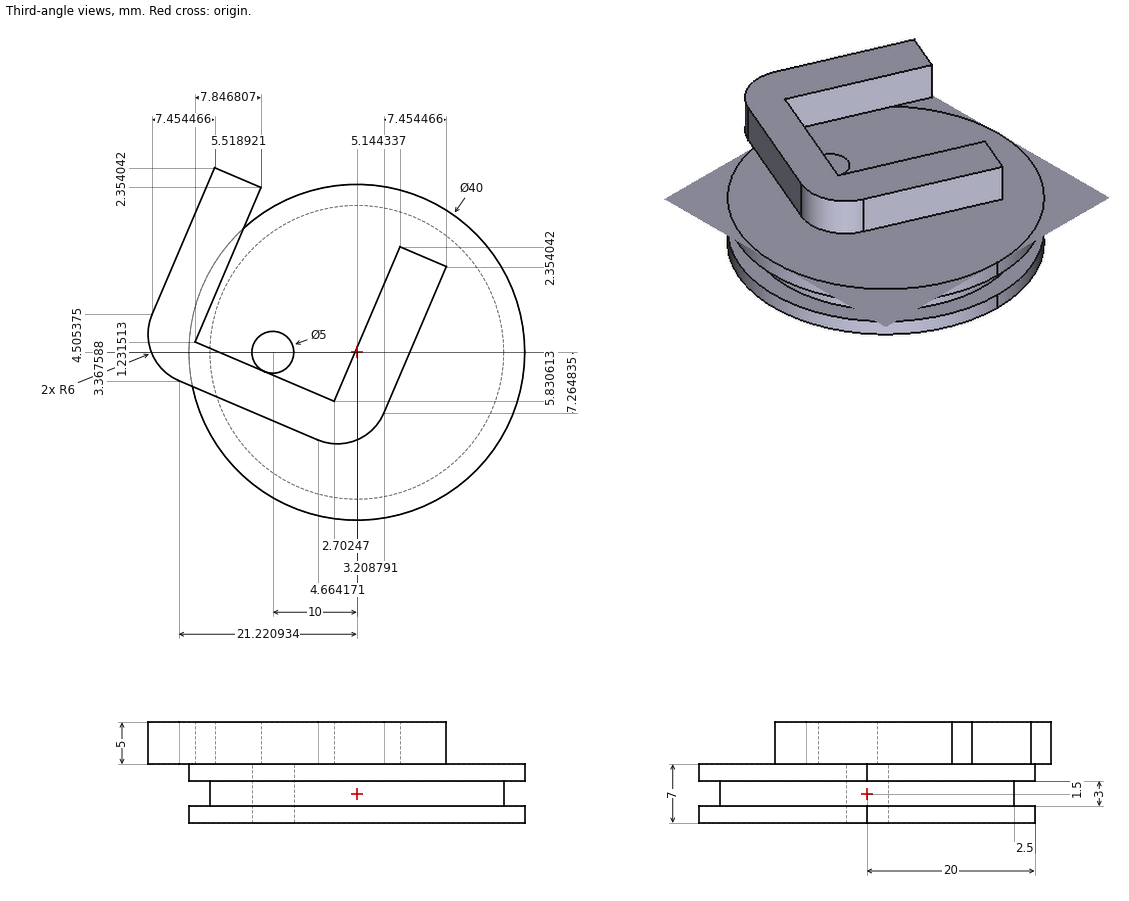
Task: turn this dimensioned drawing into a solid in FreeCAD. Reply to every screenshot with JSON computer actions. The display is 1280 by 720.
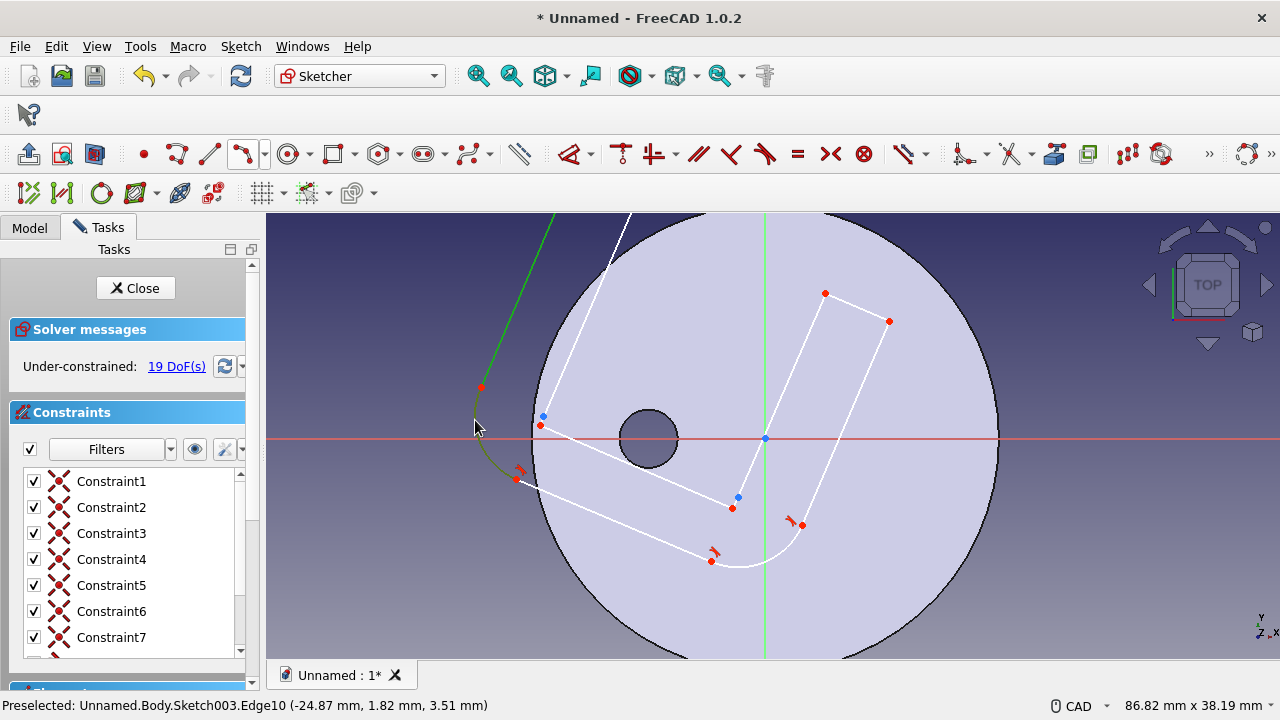
{"action": "left_click", "coordinate": [765, 154]}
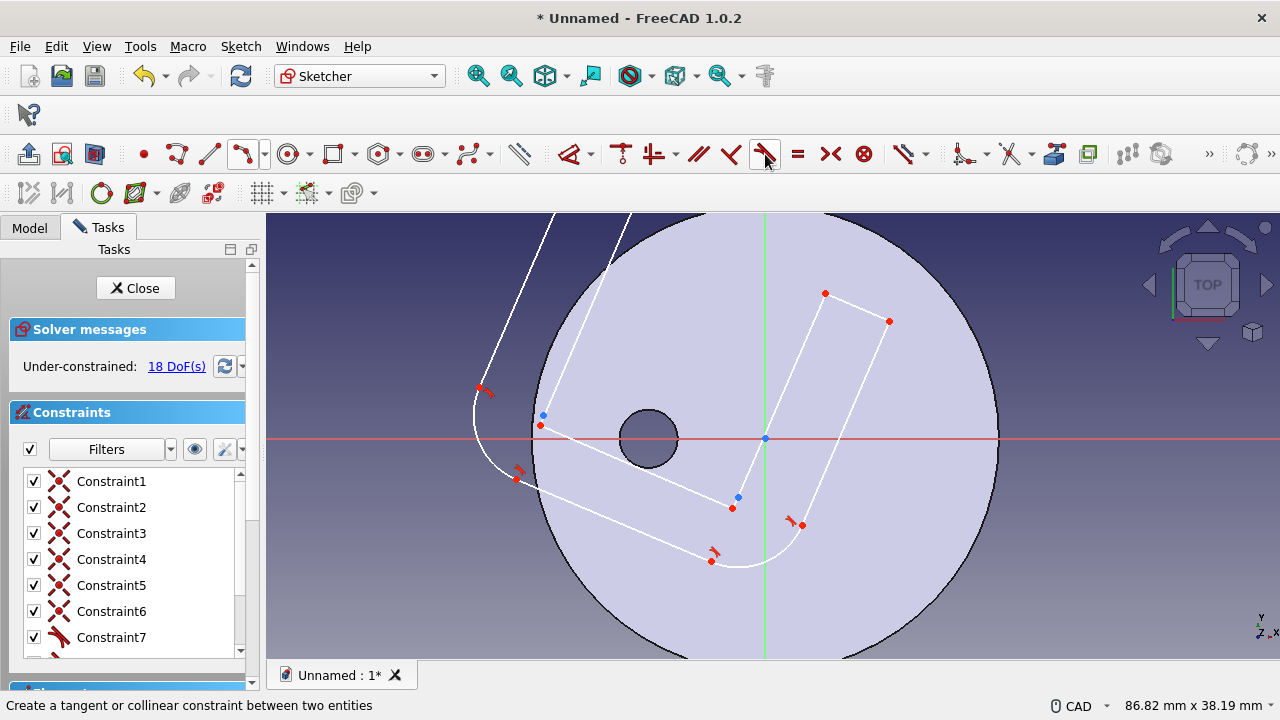
{"action": "left_click", "coordinate": [743, 567]}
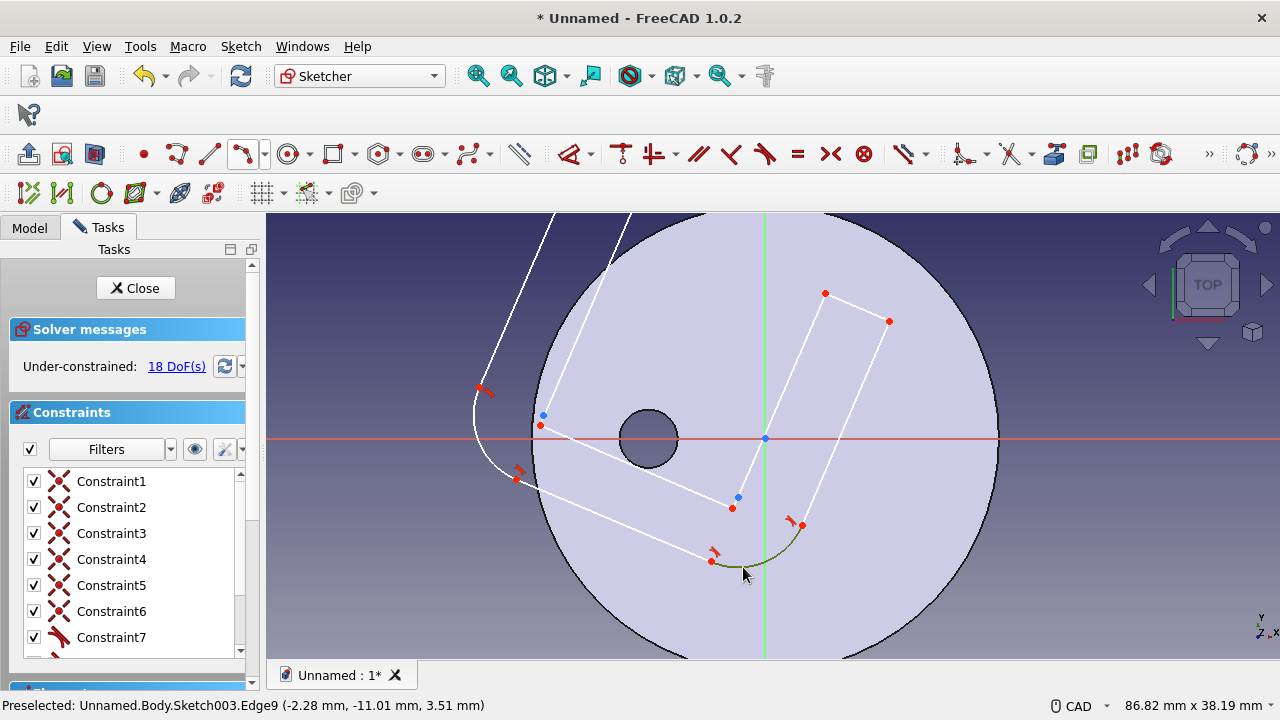
{"action": "left_click", "coordinate": [474, 420]}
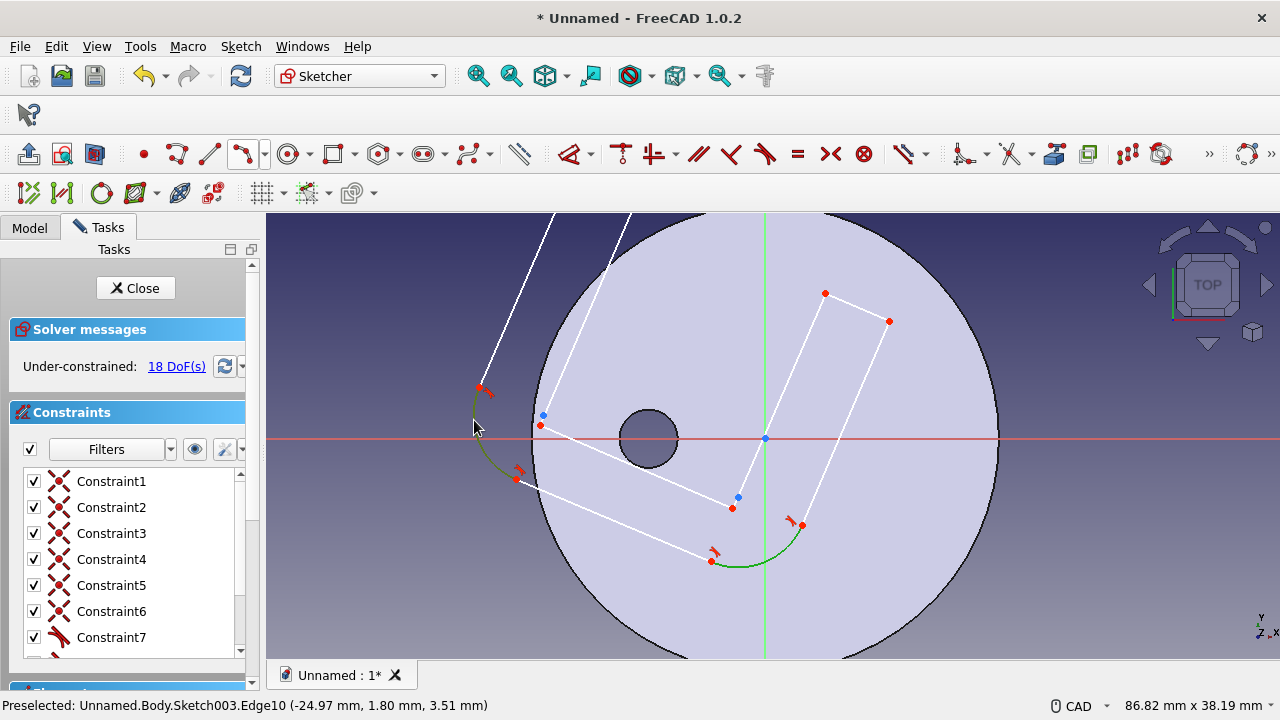
{"action": "left_click", "coordinate": [798, 154]}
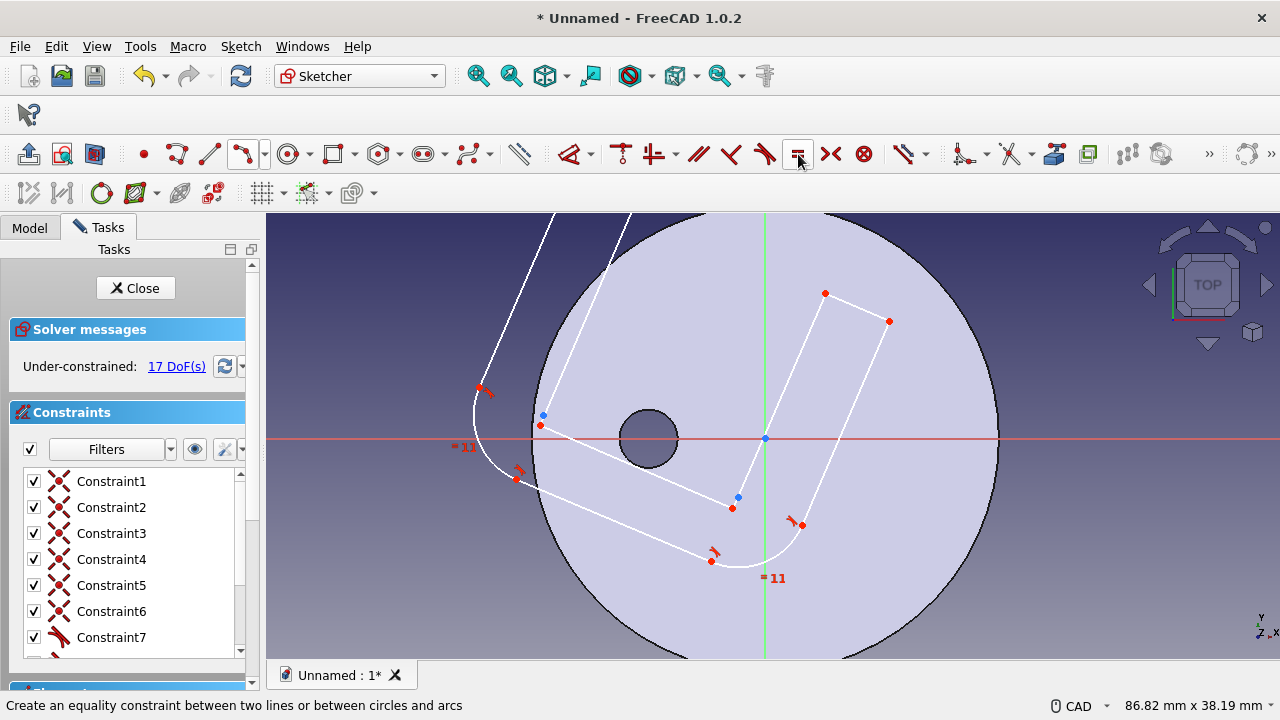
{"action": "left_click", "coordinate": [568, 154]}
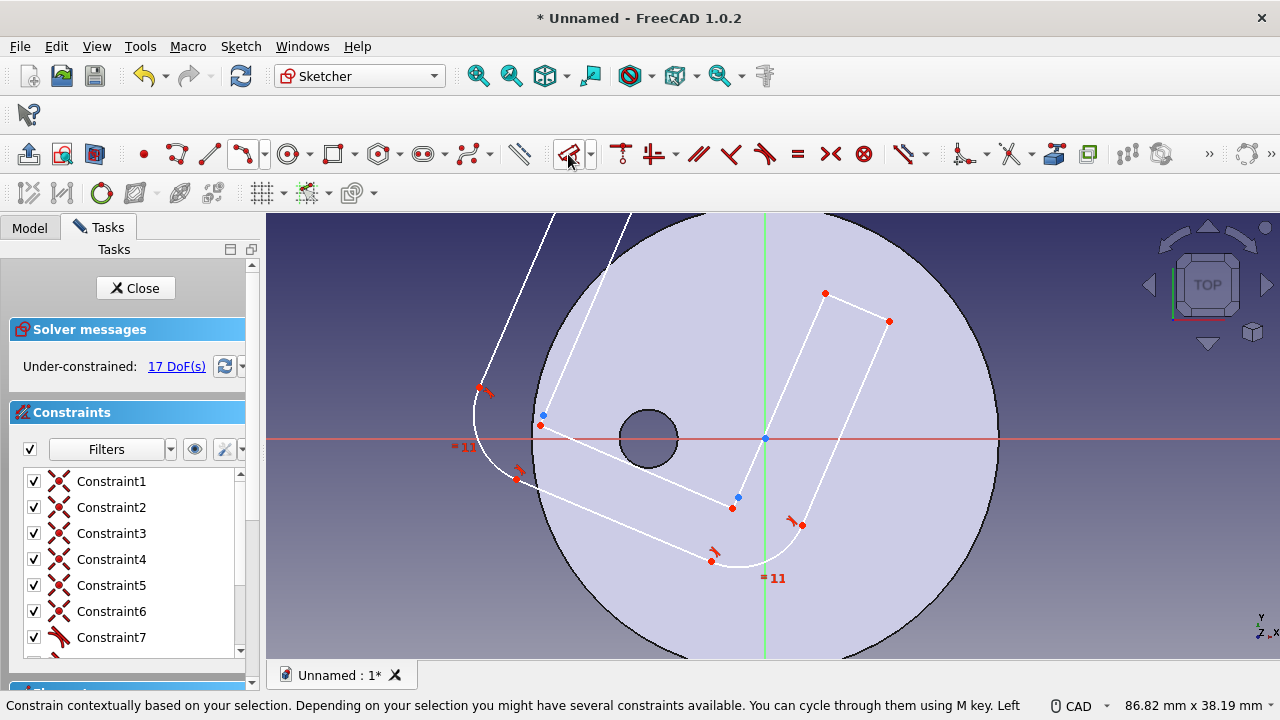
{"action": "left_click", "coordinate": [743, 567]}
{"action": "left_click", "coordinate": [745, 599]}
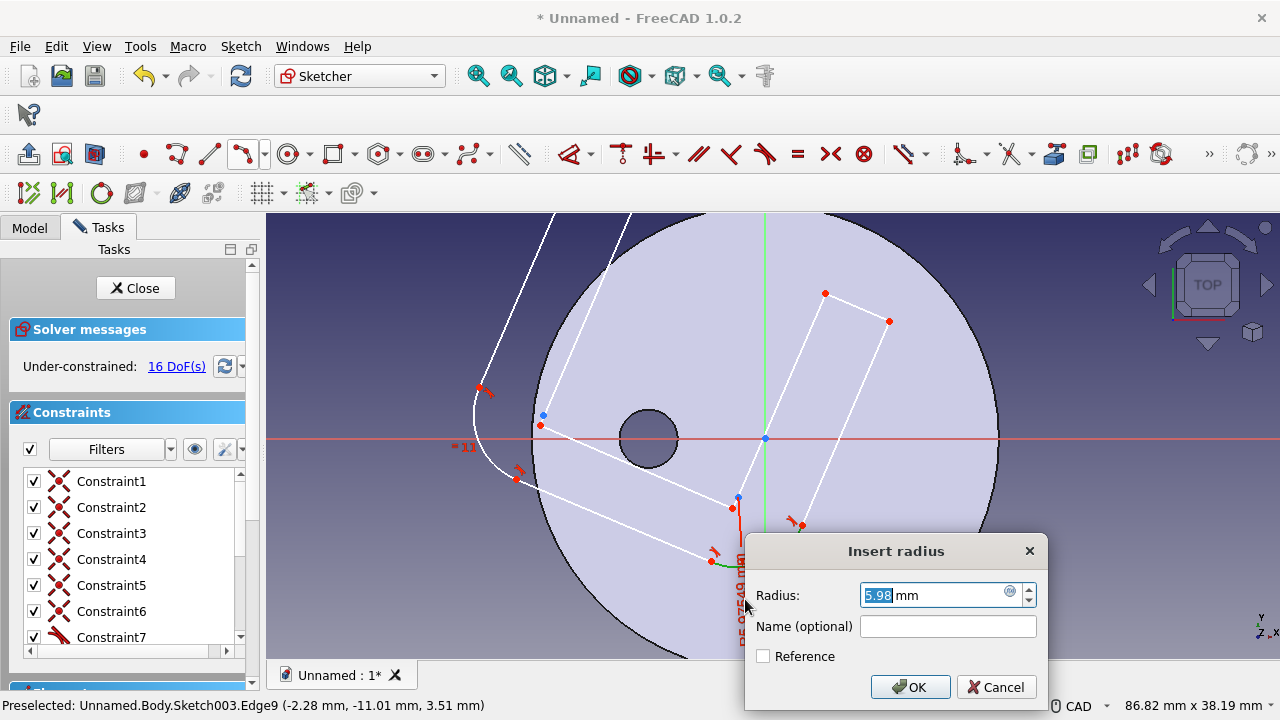
{"action": "type", "text": "6"}
{"action": "key", "text": "Return"}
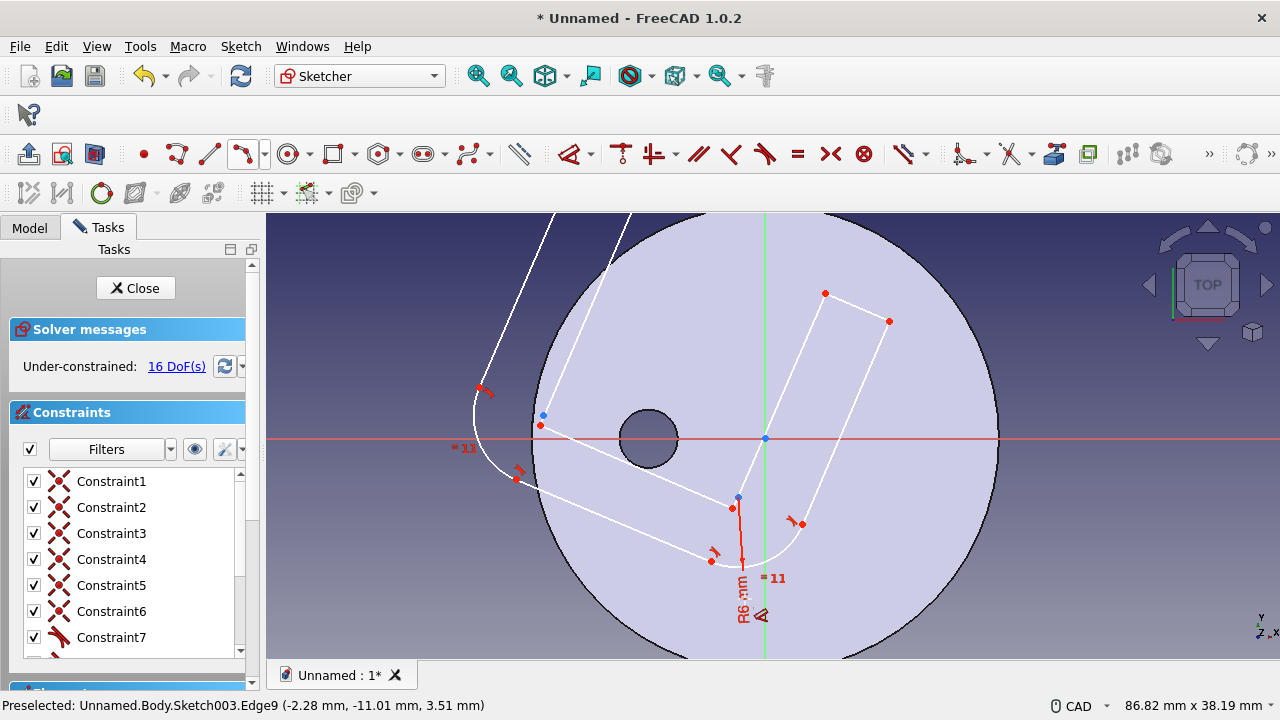
{"action": "scroll", "coordinate": [733, 509], "scroll_direction": "up", "scroll_amount": 2}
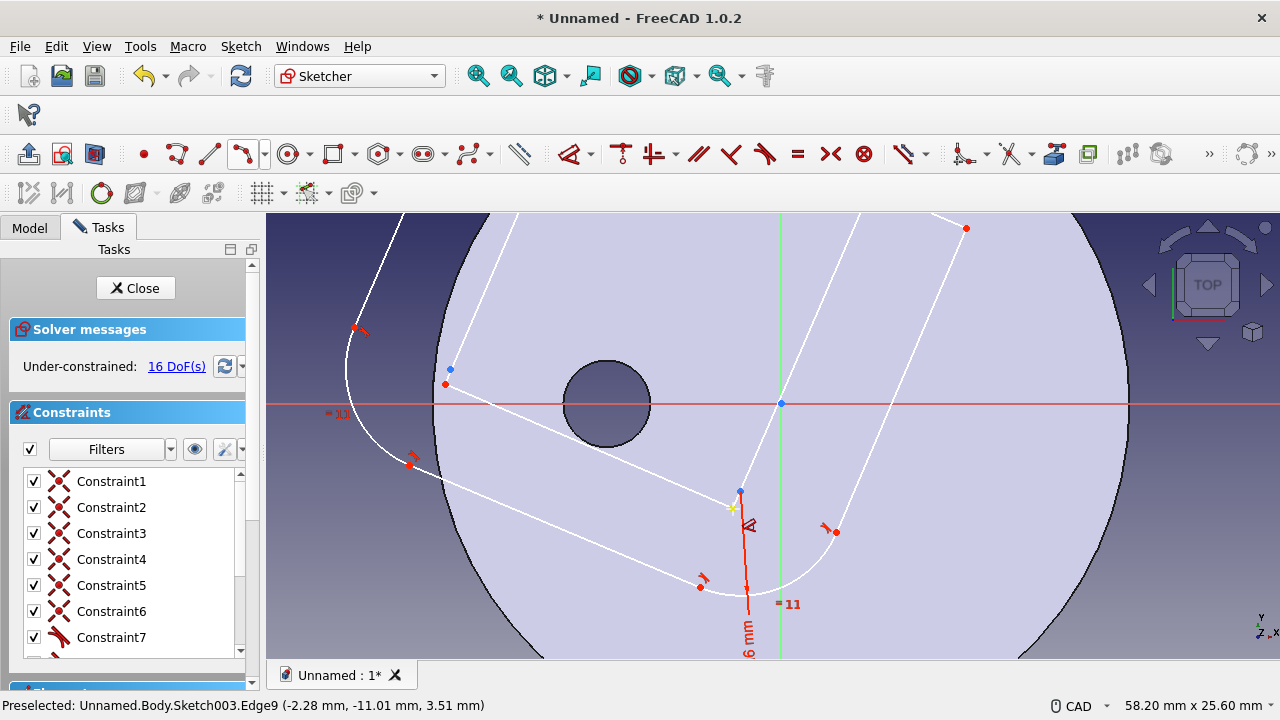
{"action": "left_click", "coordinate": [733, 508]}
{"action": "left_click", "coordinate": [757, 542]}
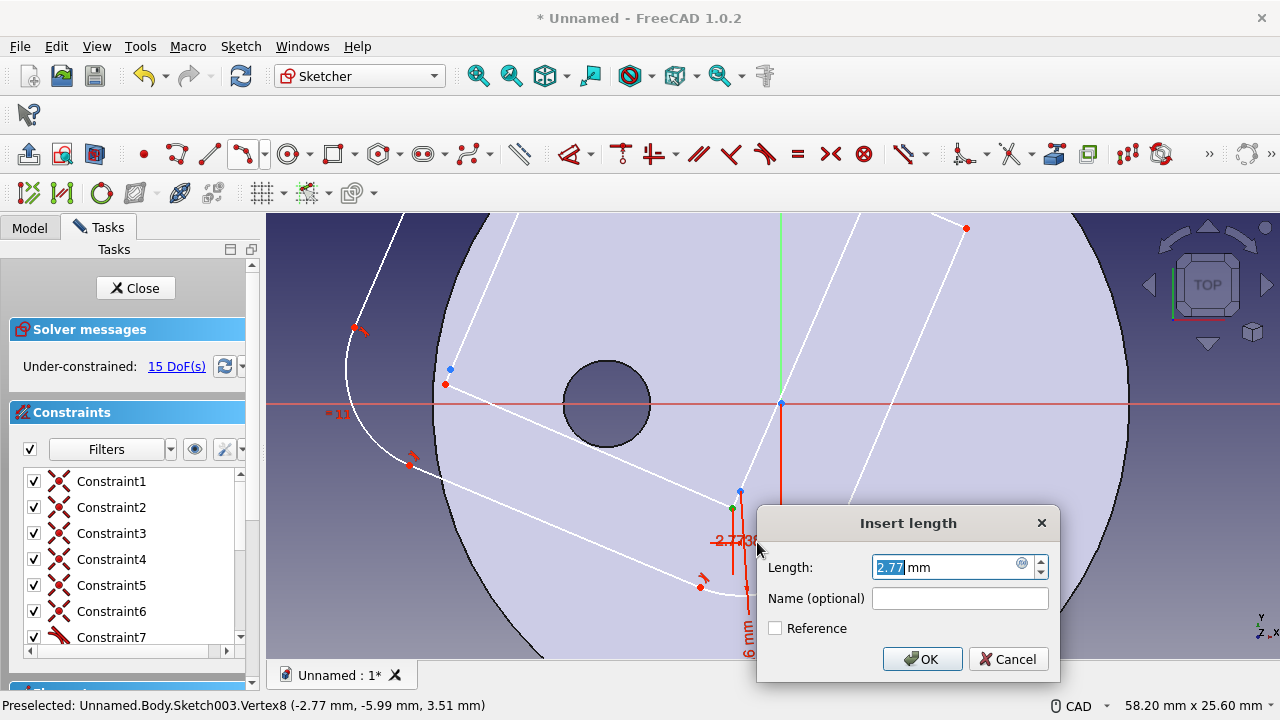
{"action": "type", "text": "2.70247"}
{"action": "key", "text": "Return"}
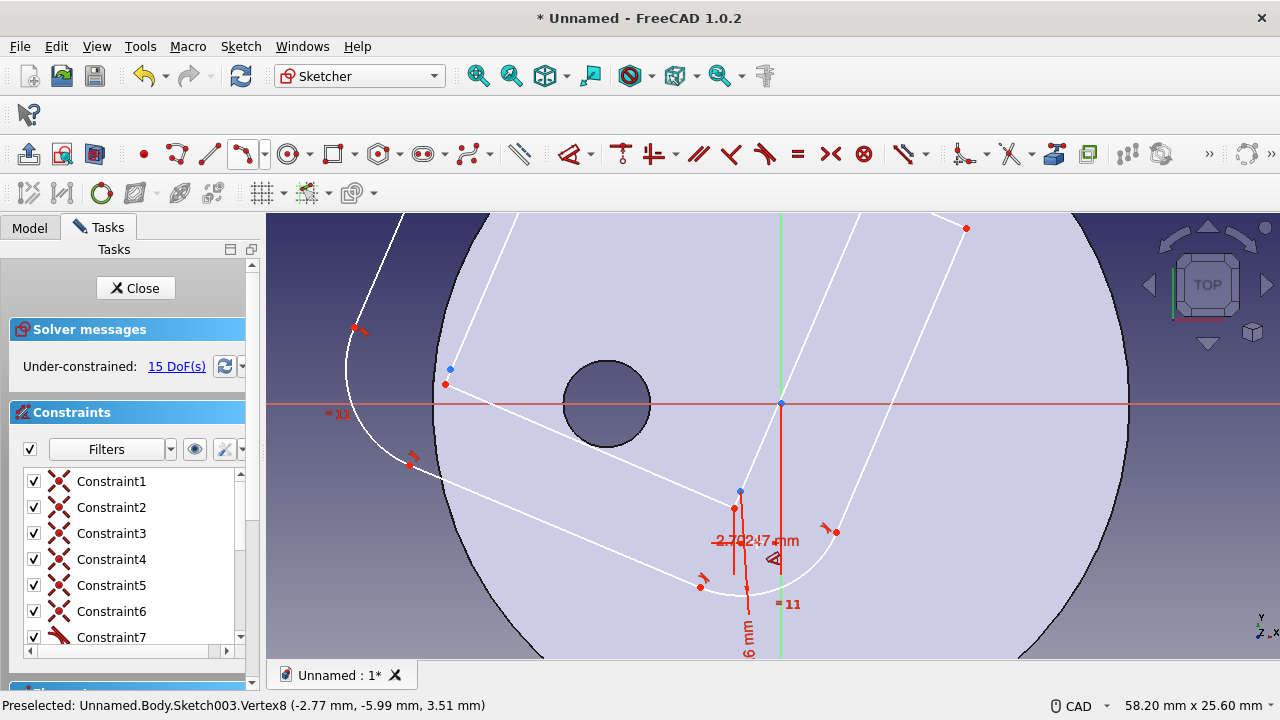
{"action": "left_click", "coordinate": [410, 465]}
{"action": "left_click", "coordinate": [376, 420]}